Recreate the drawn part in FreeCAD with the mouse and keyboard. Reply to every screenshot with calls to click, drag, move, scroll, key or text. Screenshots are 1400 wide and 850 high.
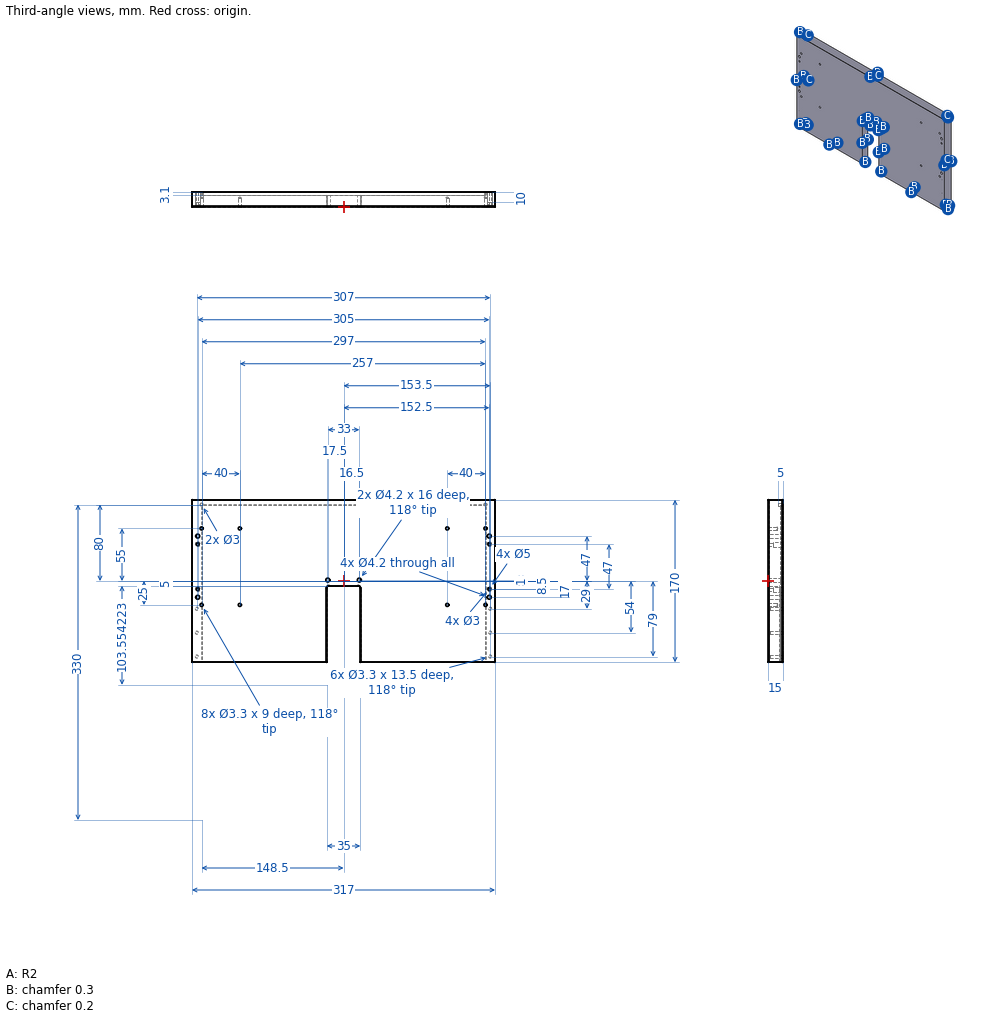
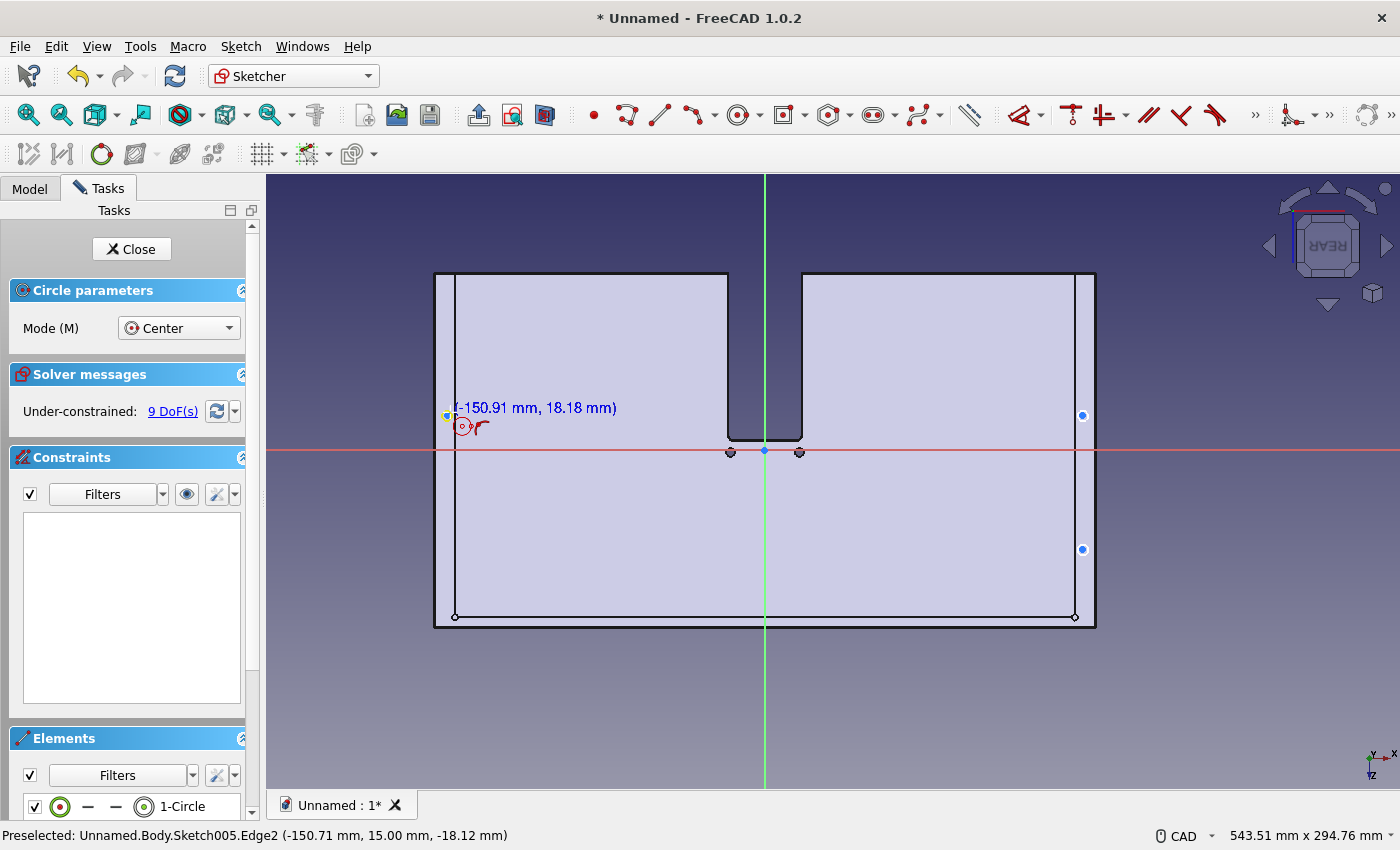
scroll(447, 549, up, 9)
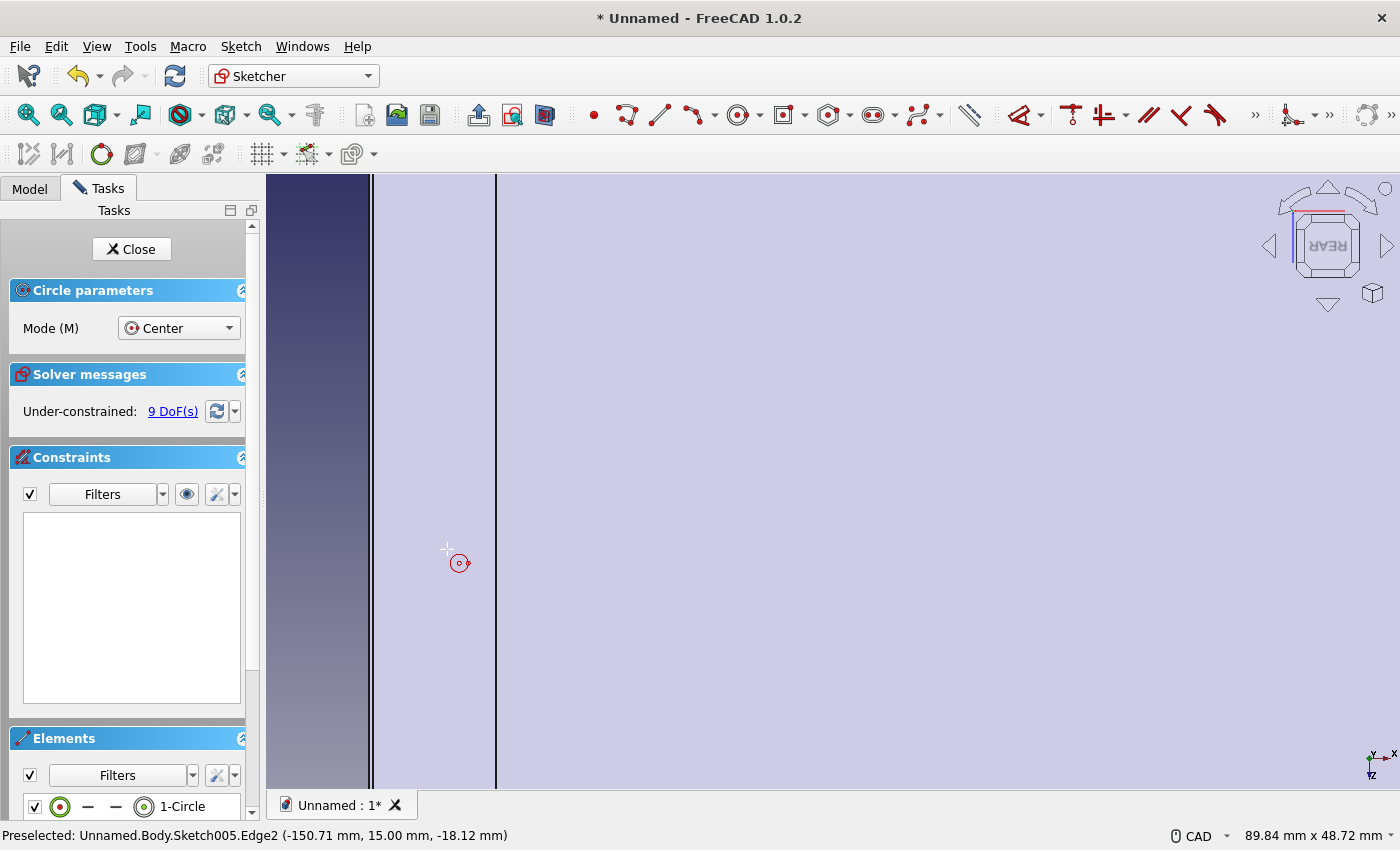
scroll(447, 549, down, 9)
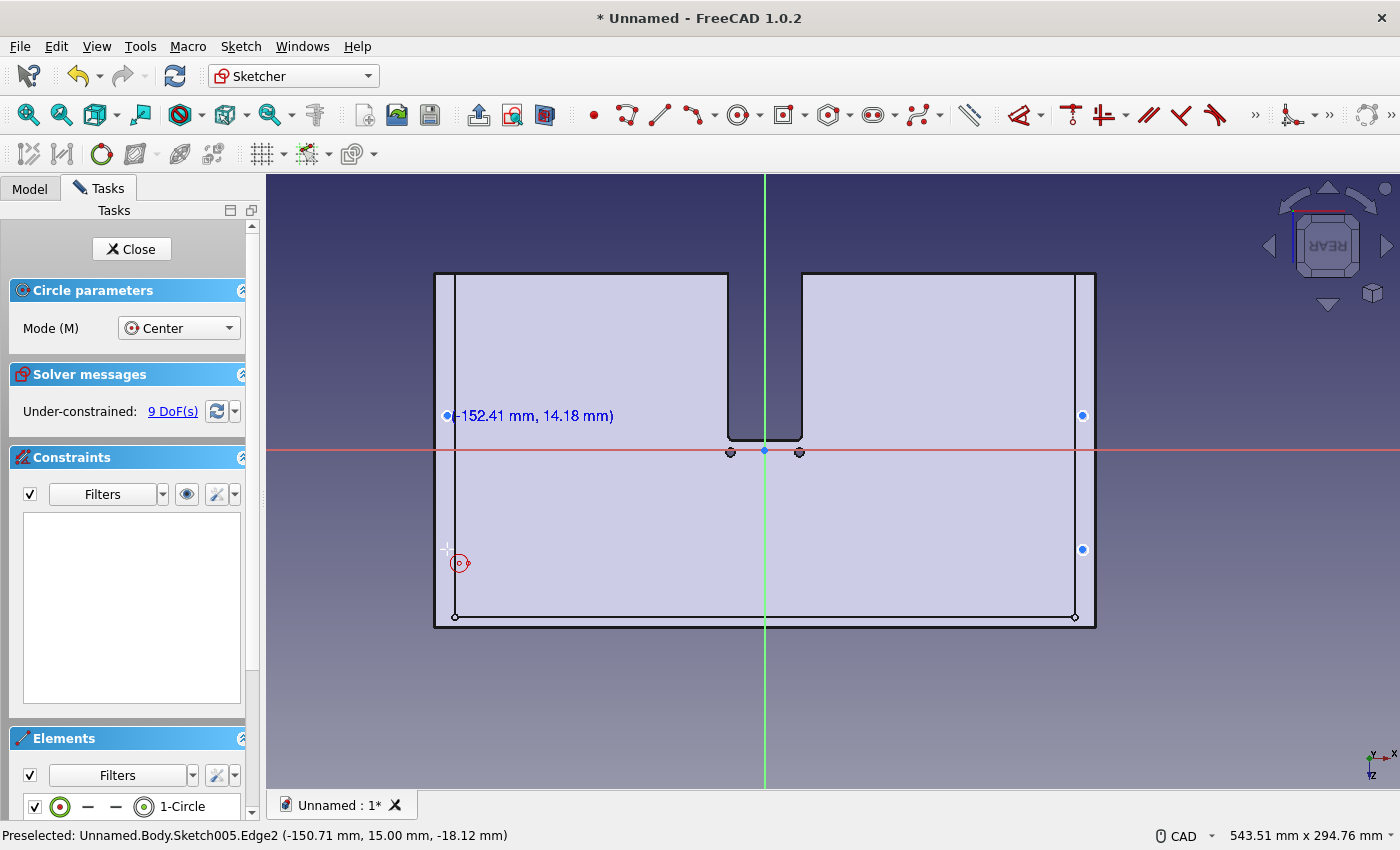
click(447, 549)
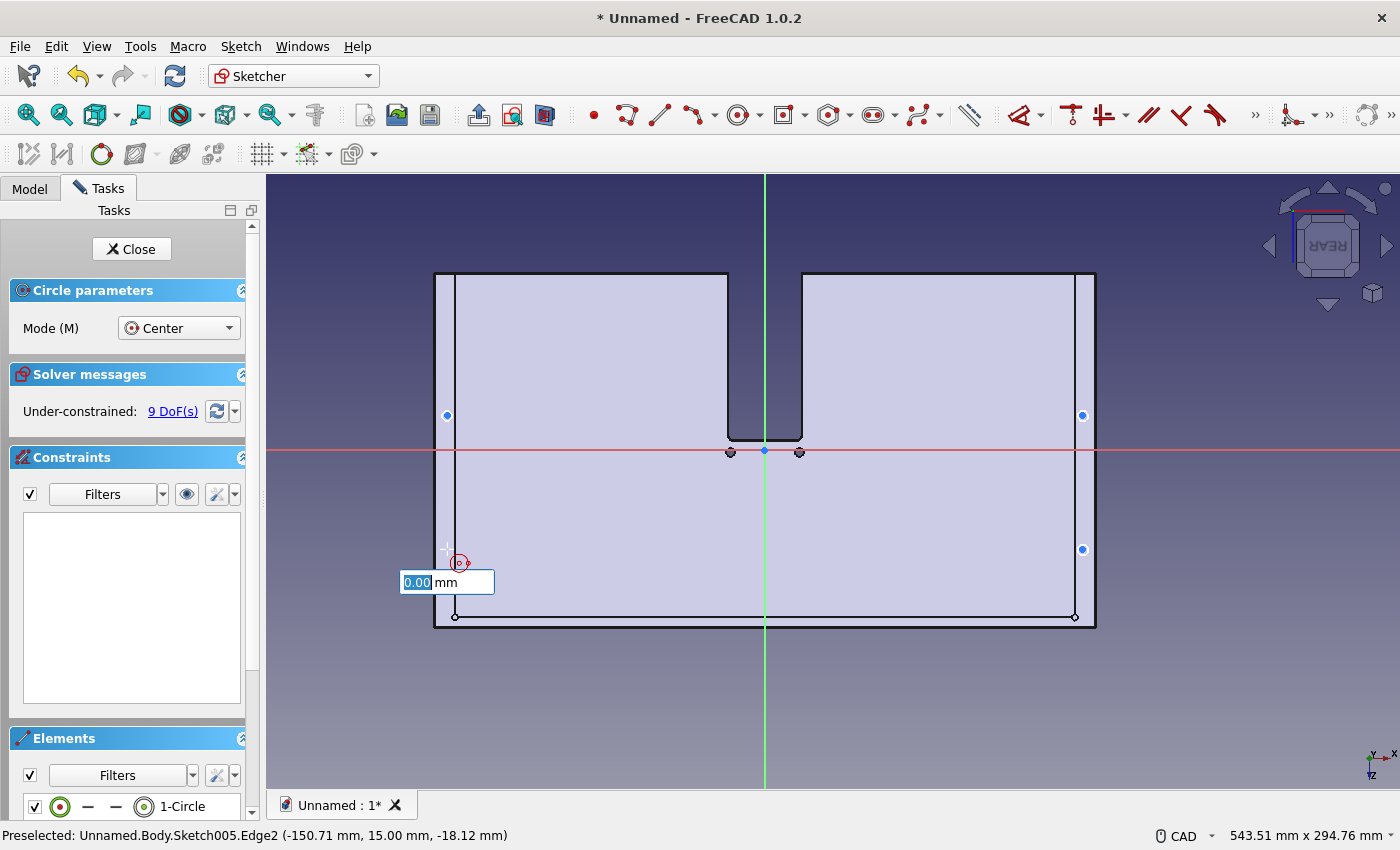
scroll(450, 545, up, 7)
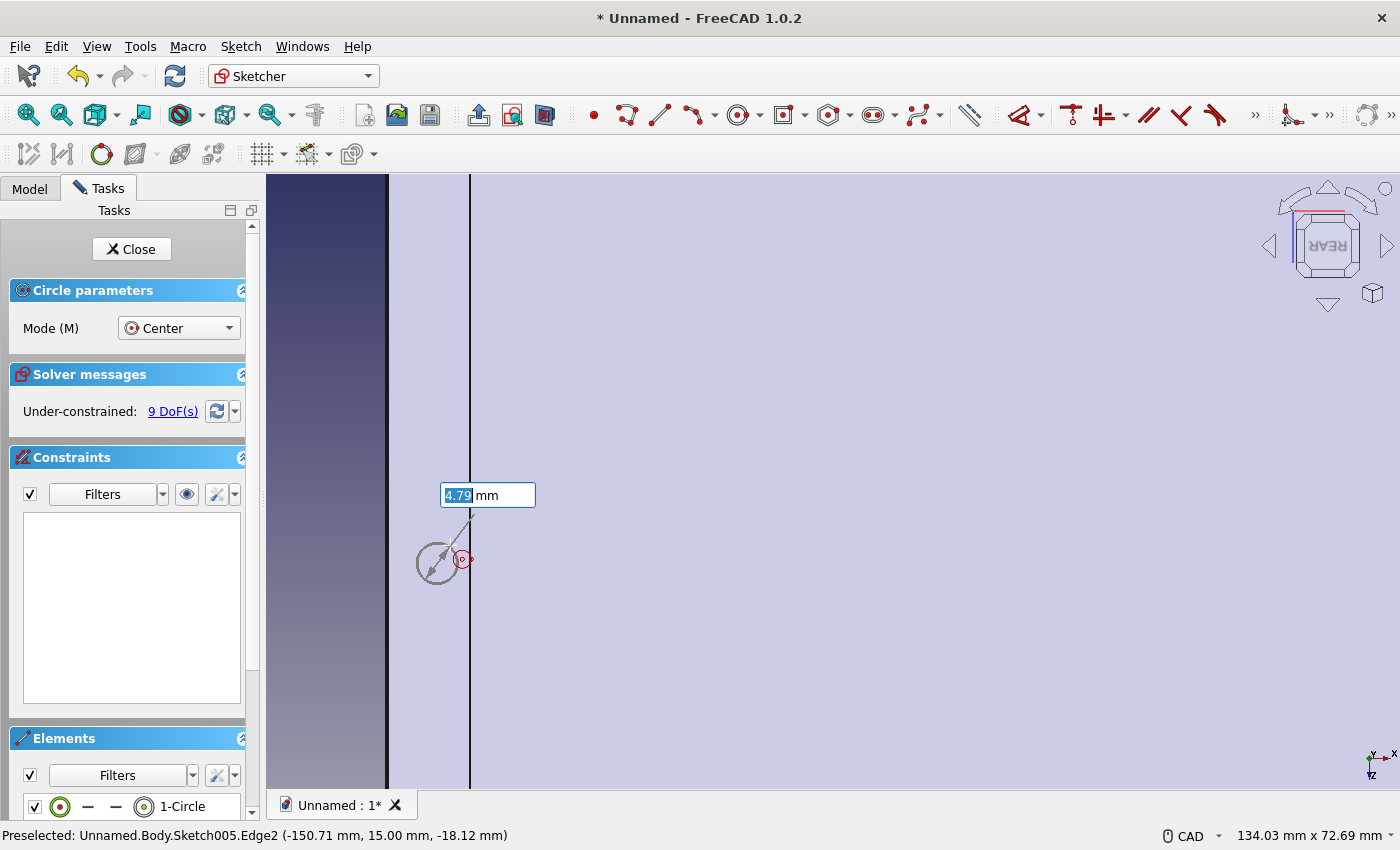
click(449, 545)
key(Escape)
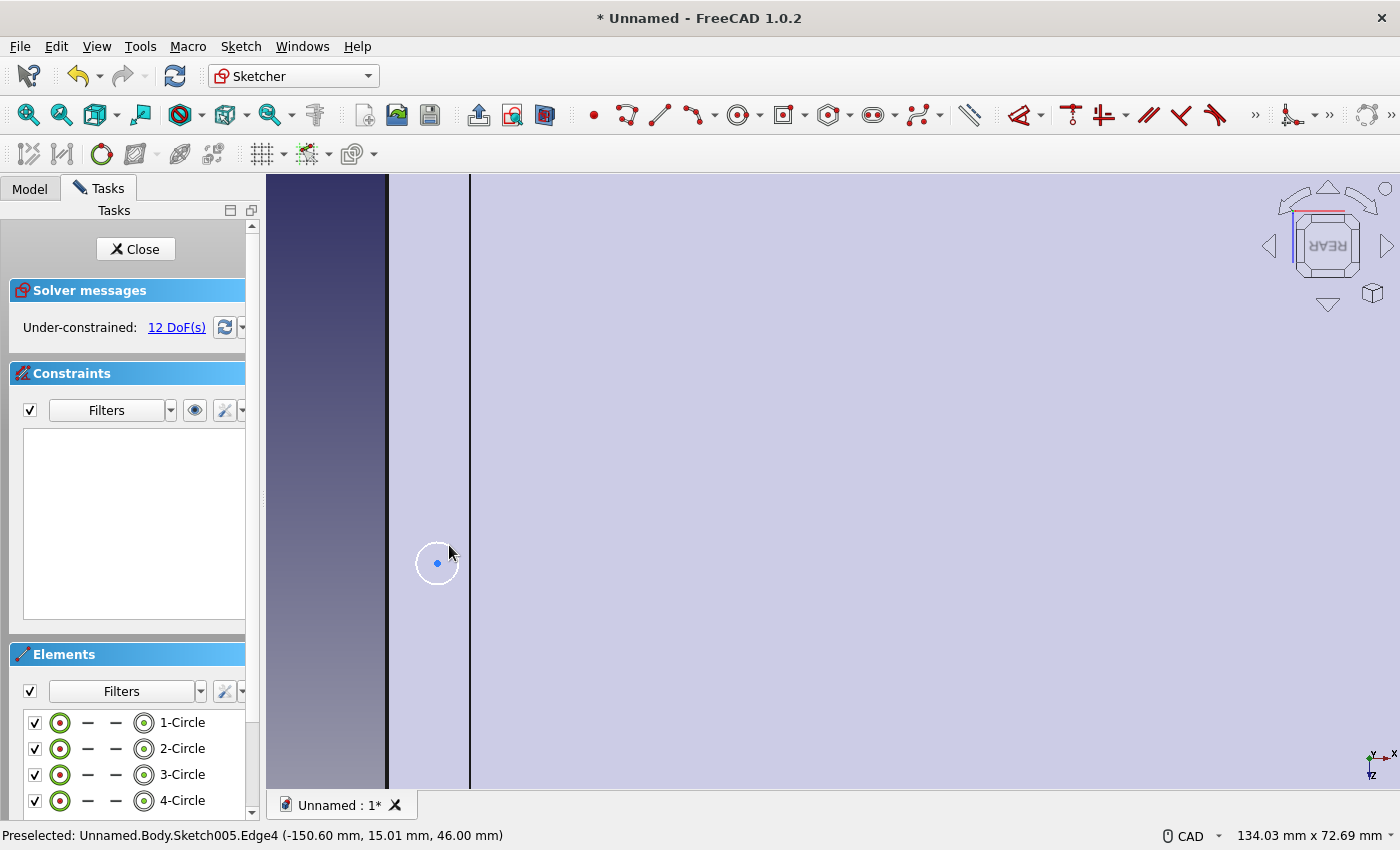
scroll(450, 545, down, 7)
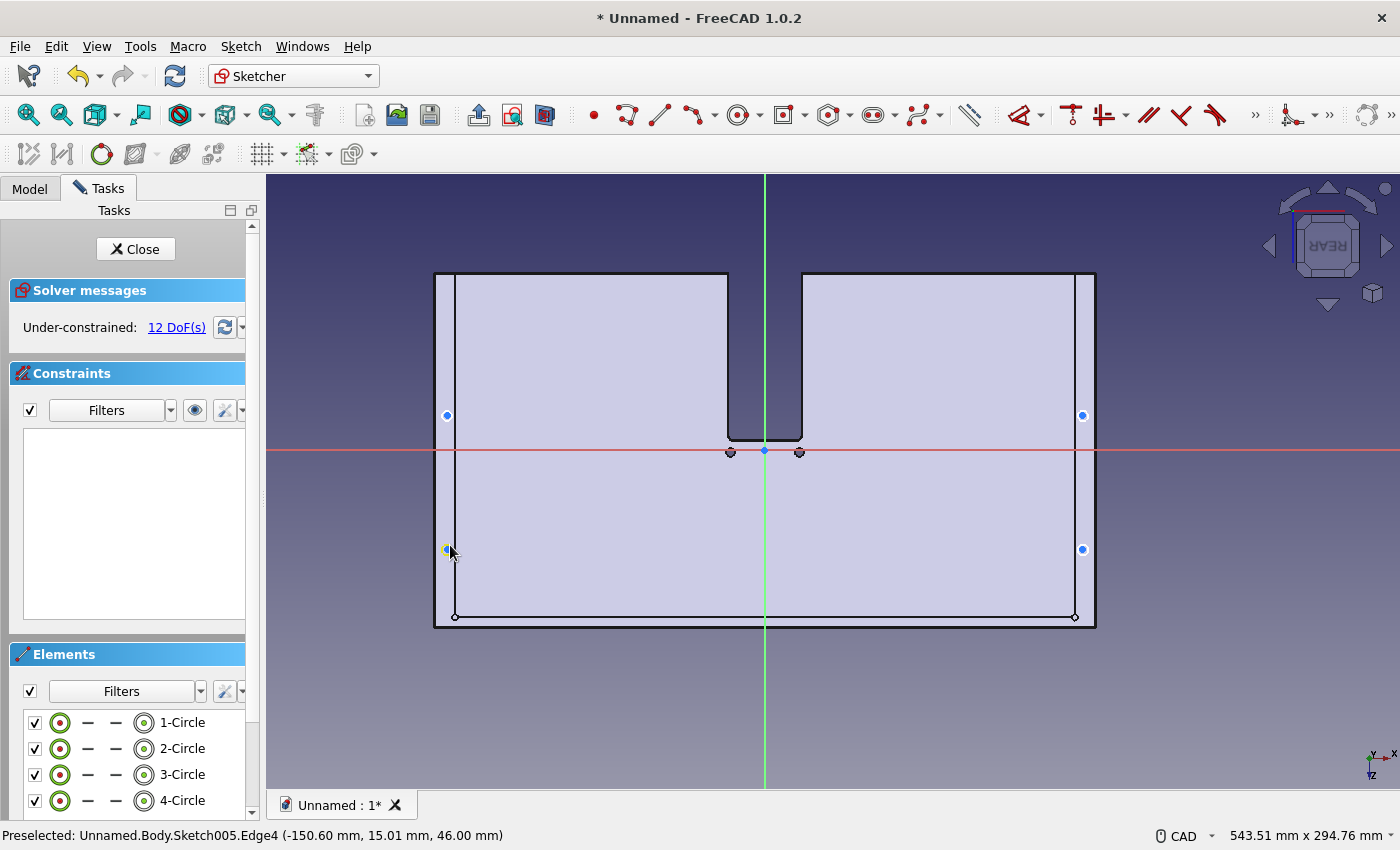
scroll(1087, 412, up, 5)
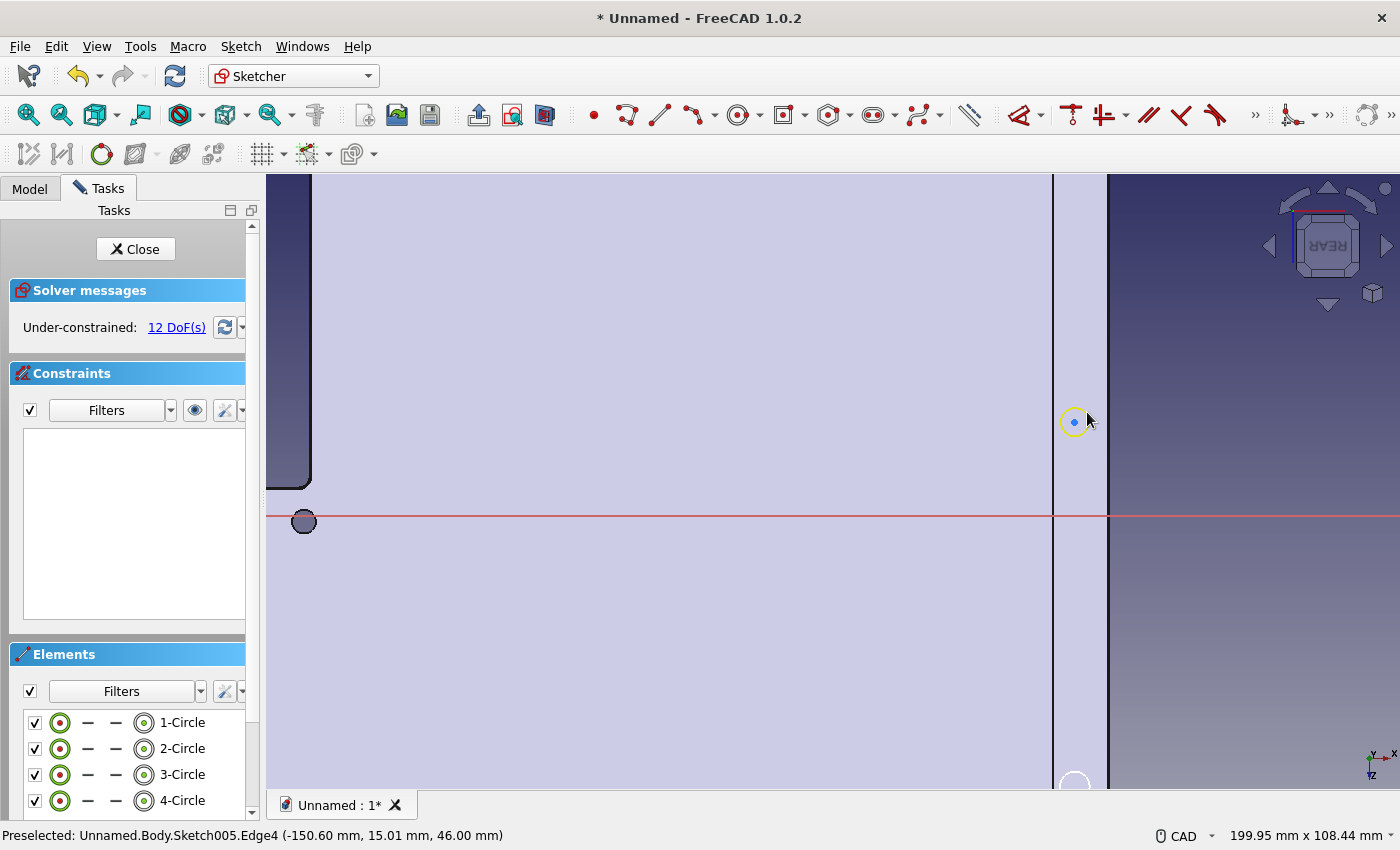
click(1085, 412)